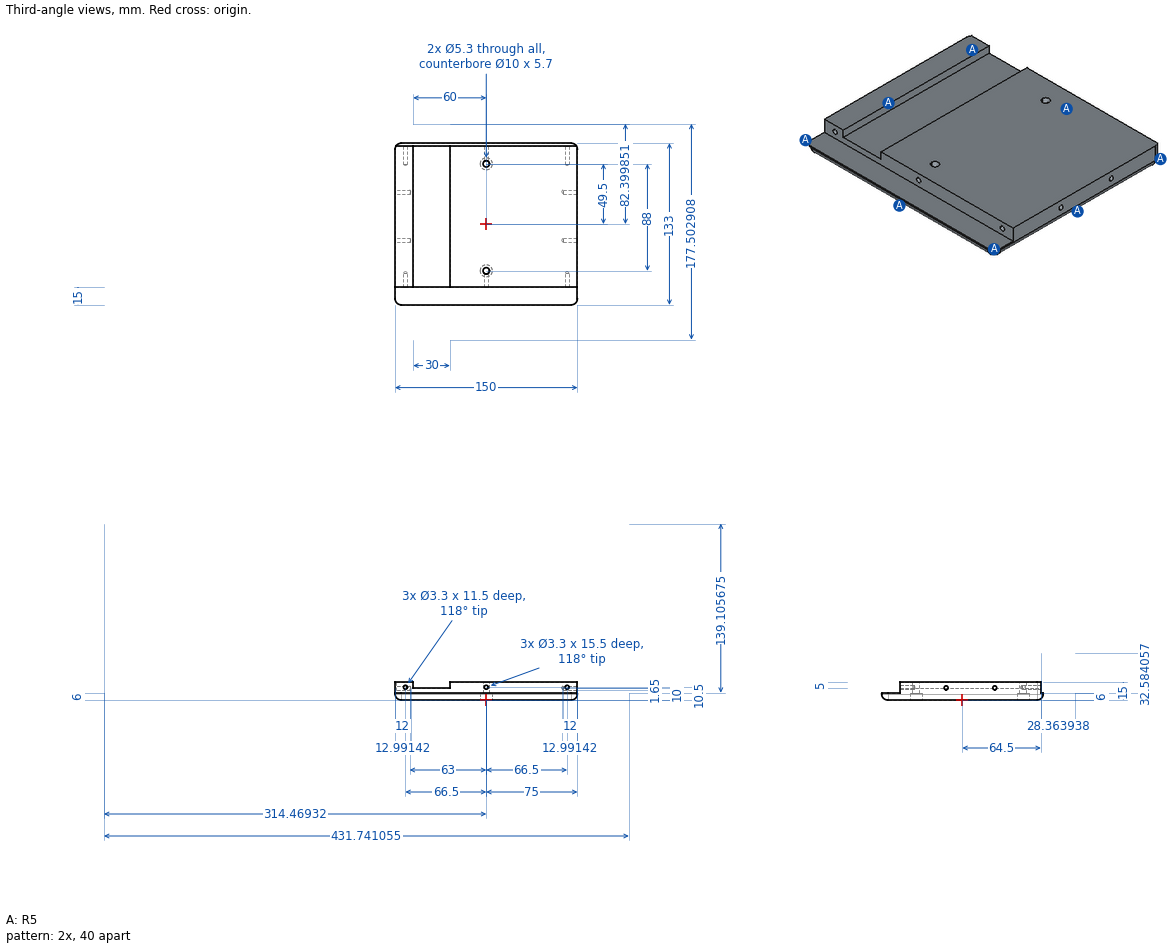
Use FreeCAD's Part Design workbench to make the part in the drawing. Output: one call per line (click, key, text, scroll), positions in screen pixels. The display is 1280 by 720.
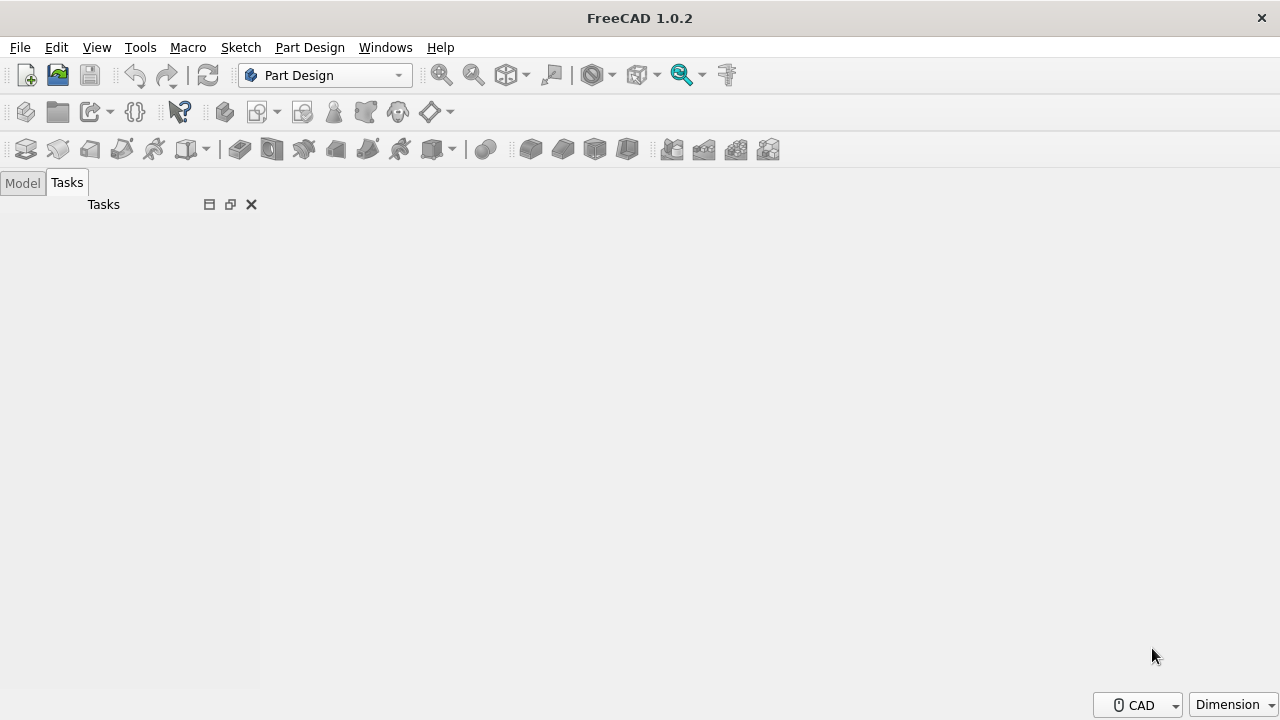
click(26, 76)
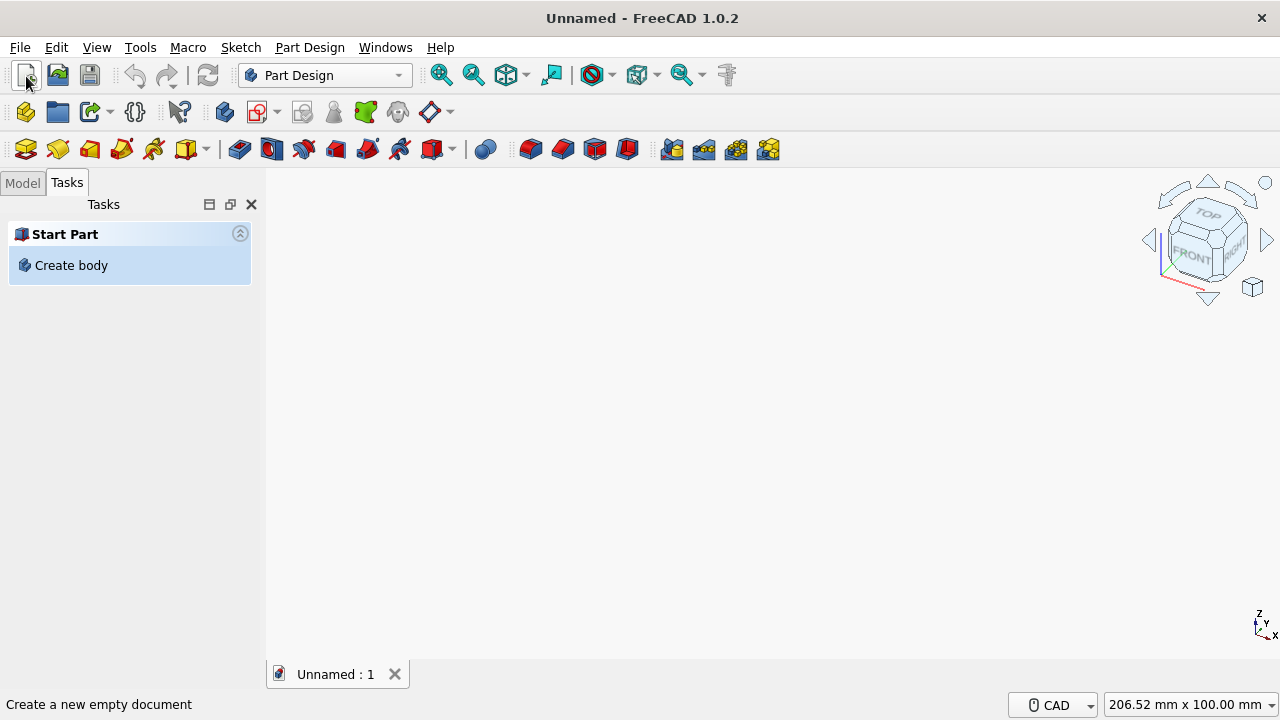
click(258, 112)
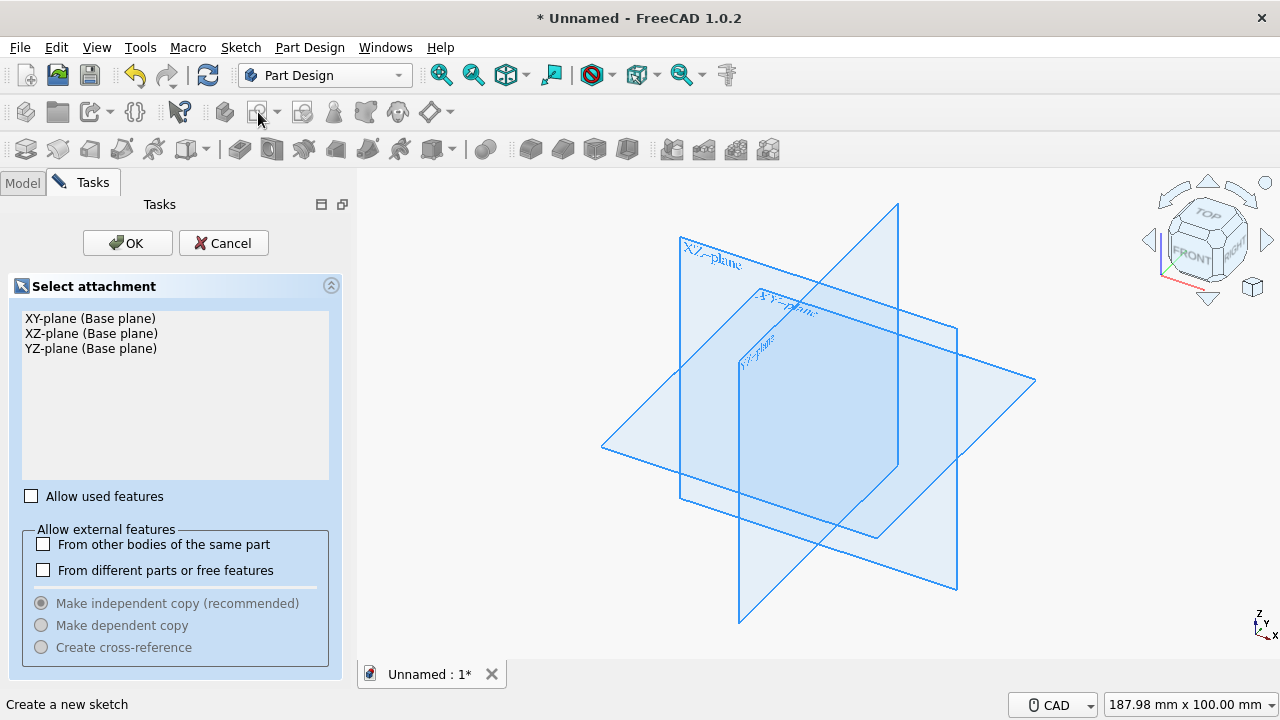
click(82, 318)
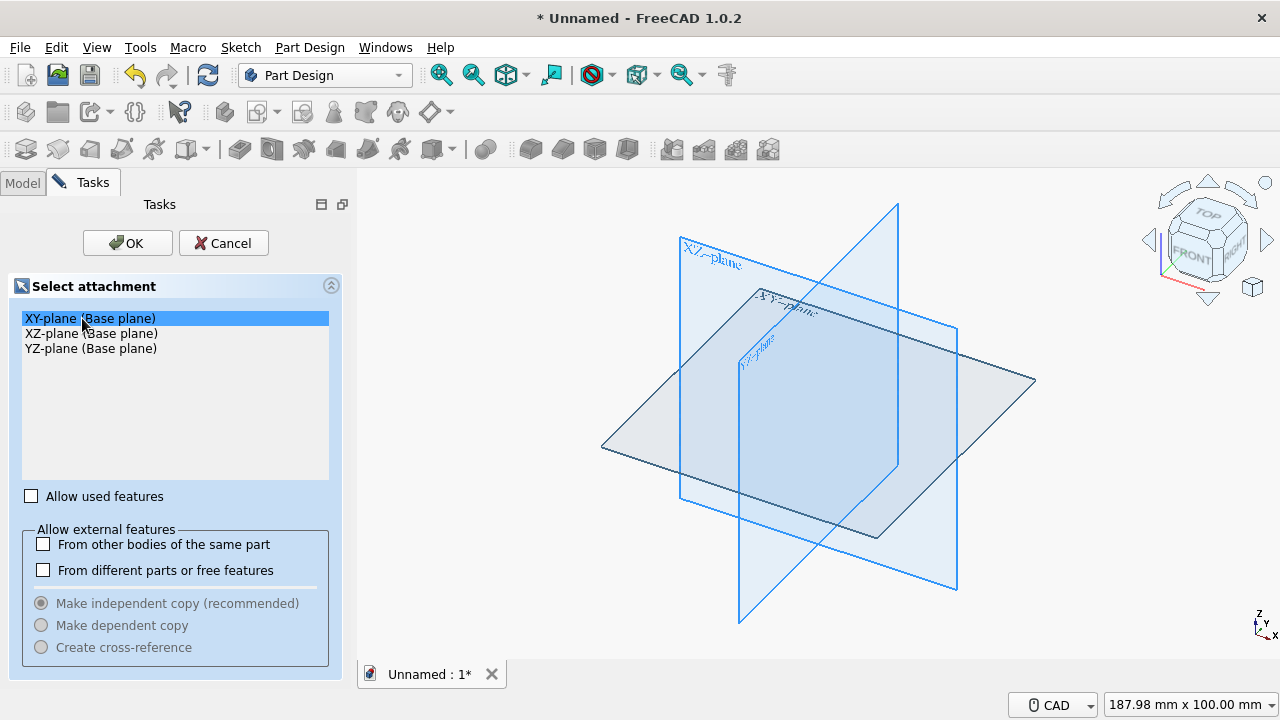
click(128, 243)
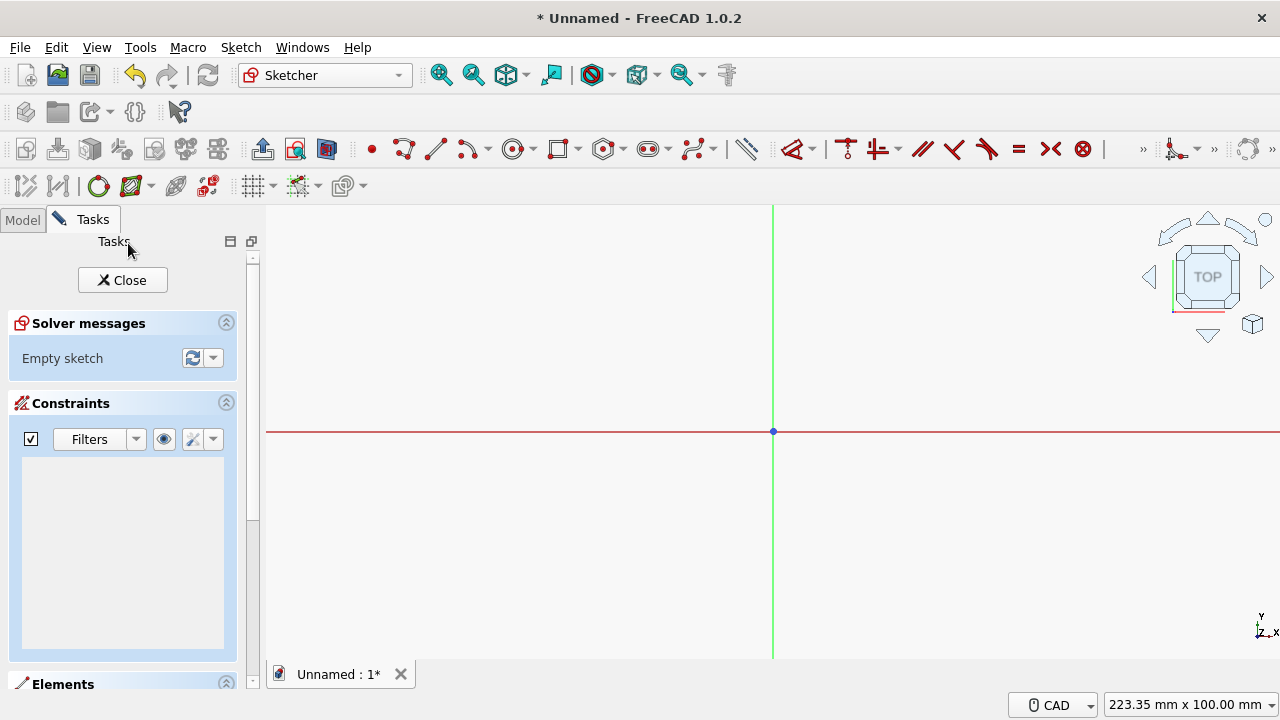
scroll(649, 432, down, 4)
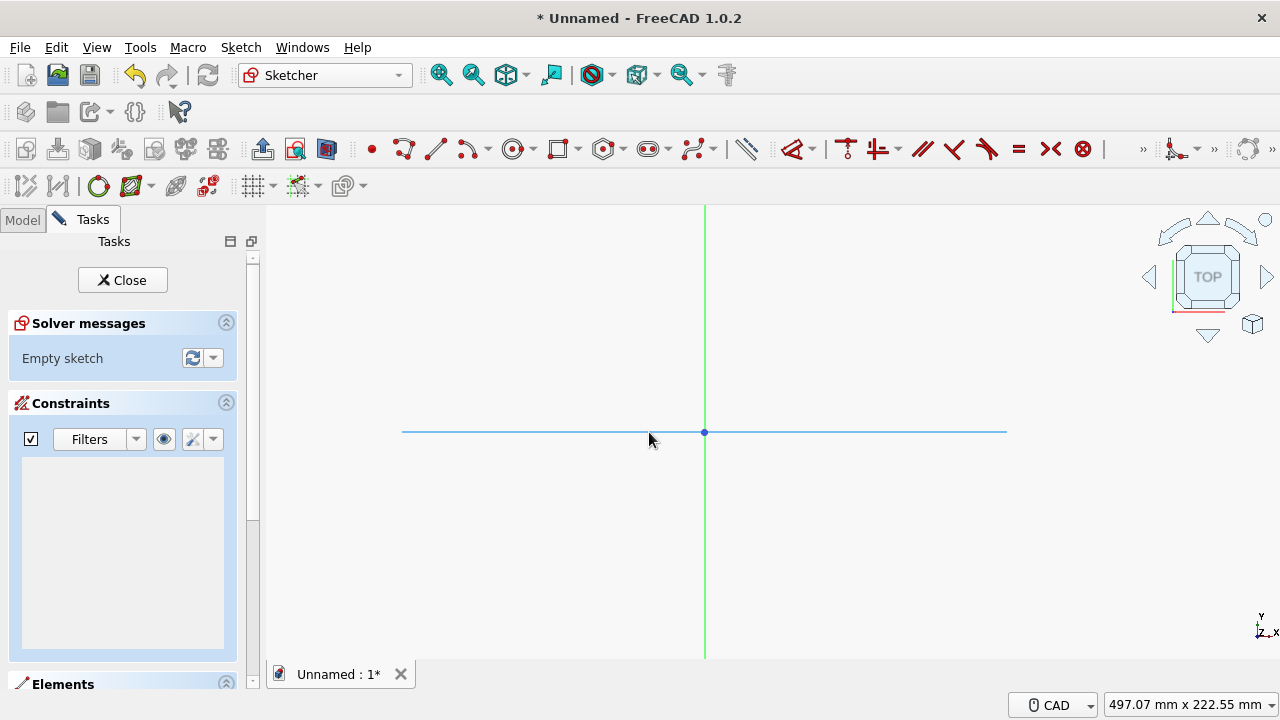
key(g)
key(v)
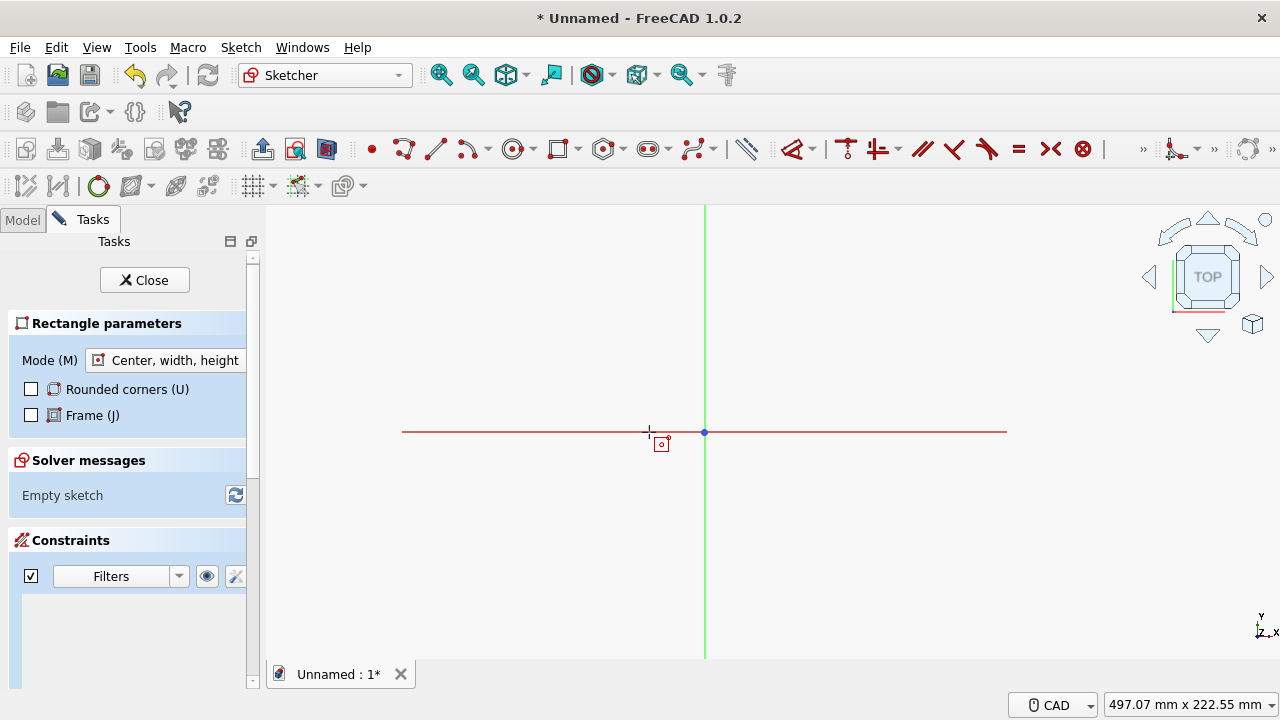
click(705, 432)
move(858, 297)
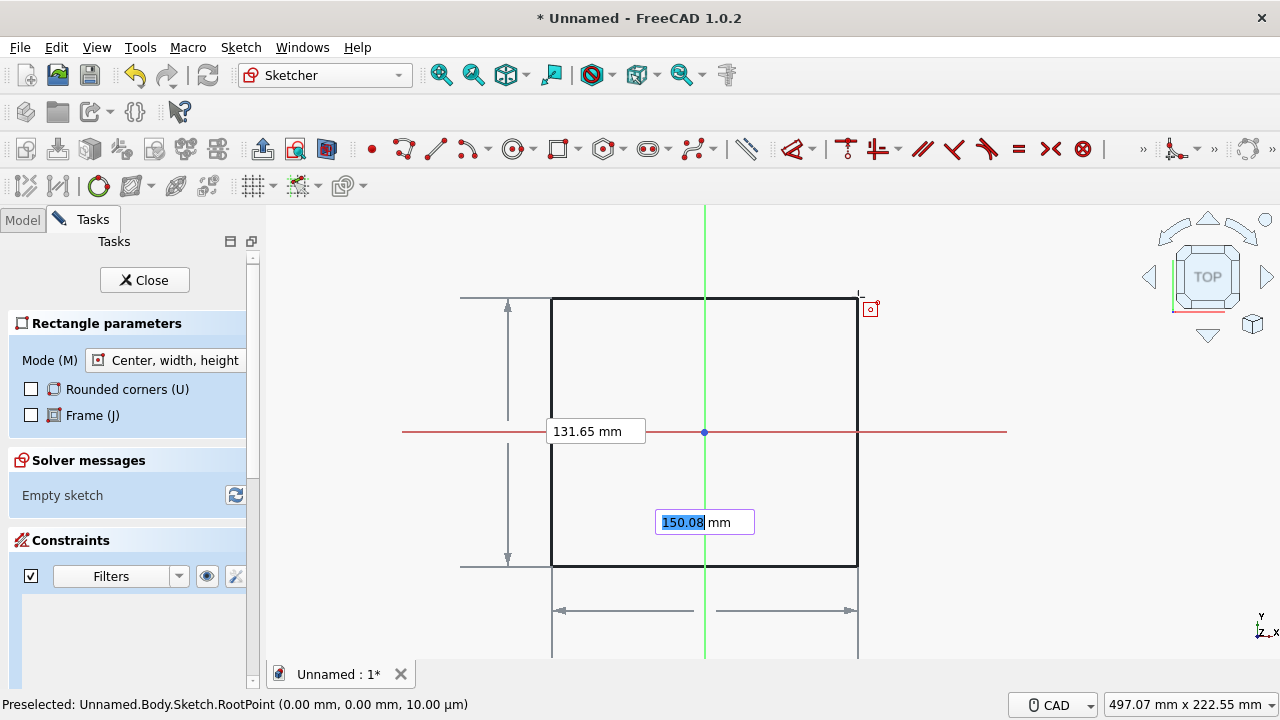
text(150)
key(Tab)
text(133)
key(Return)
key(Escape)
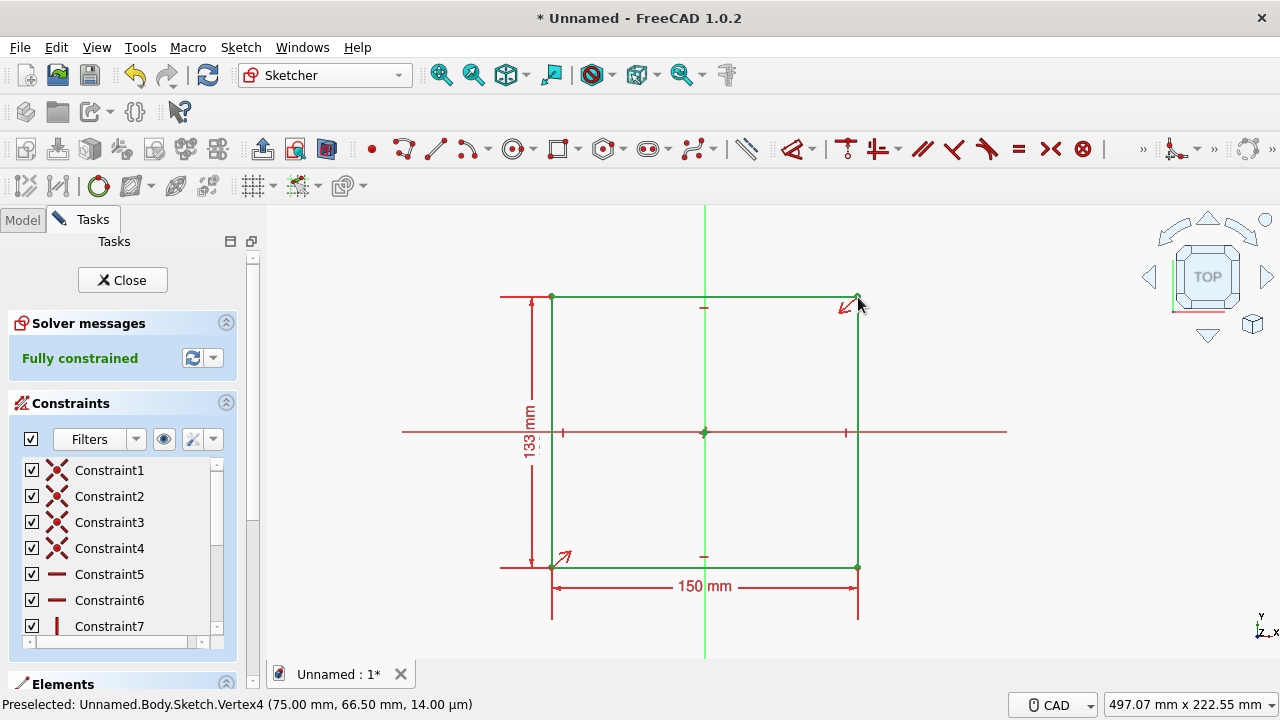
click(123, 280)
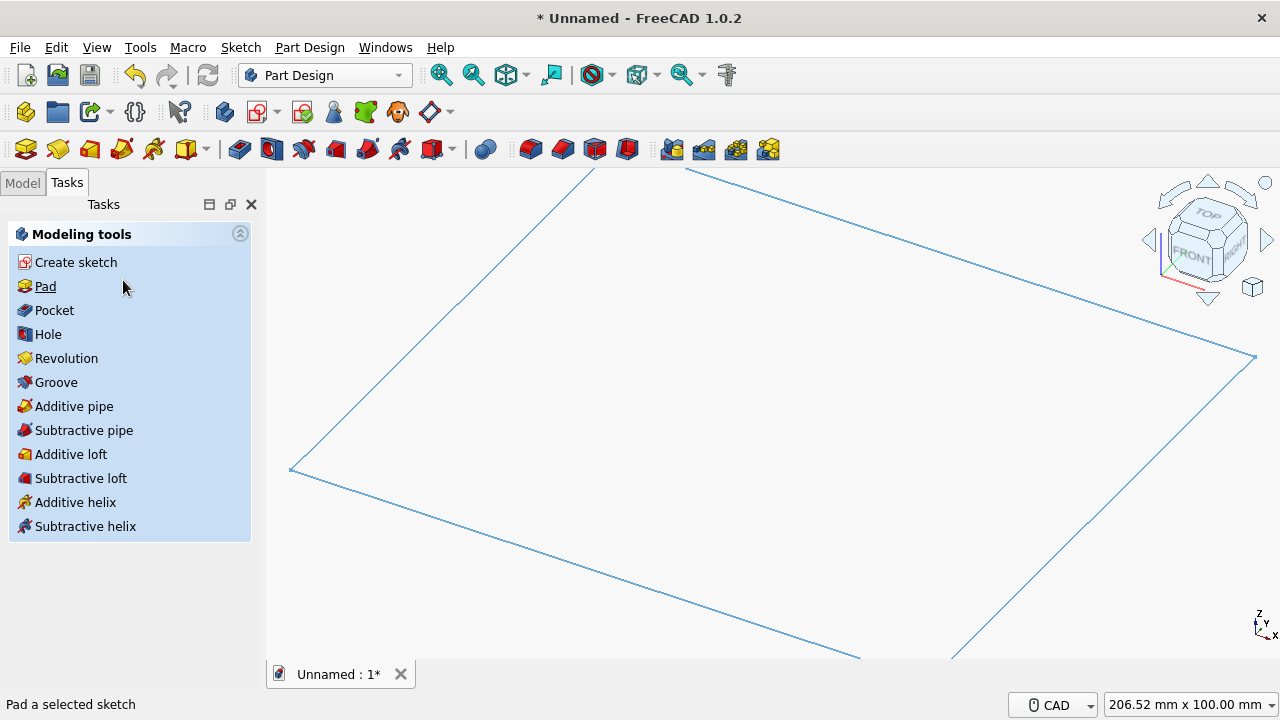
click(26, 150)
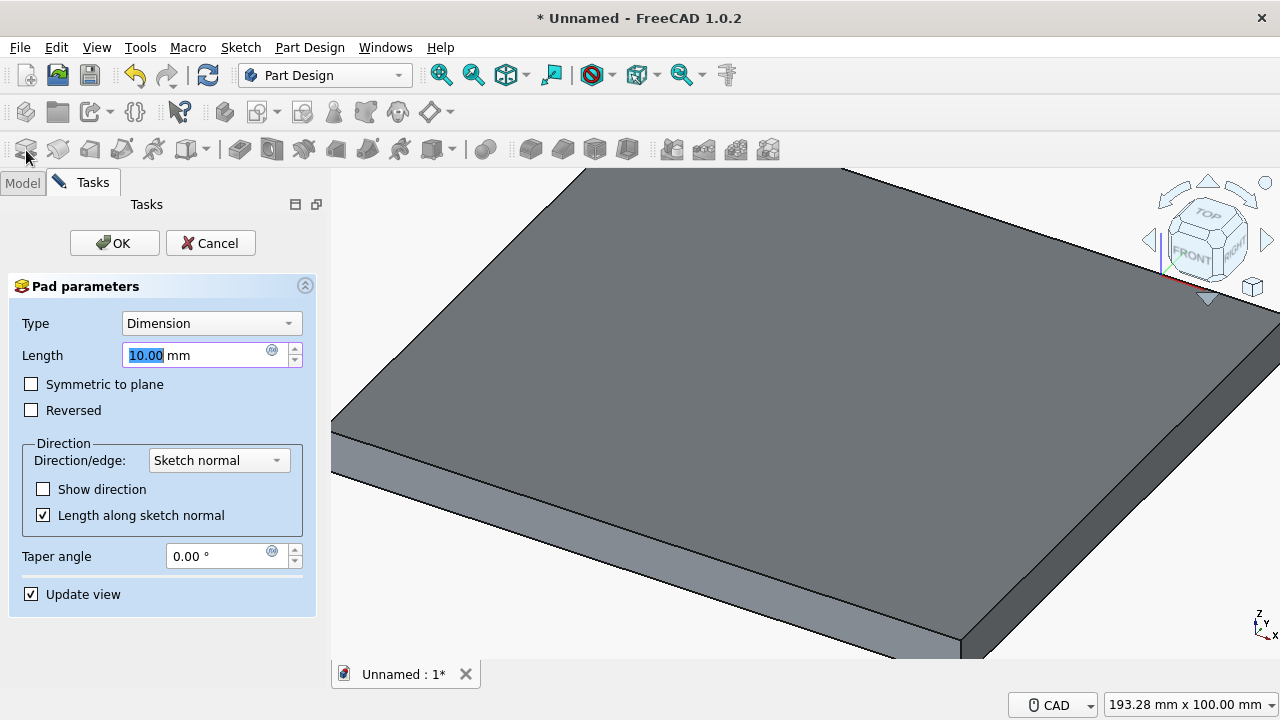
text(15)
key(Tab)